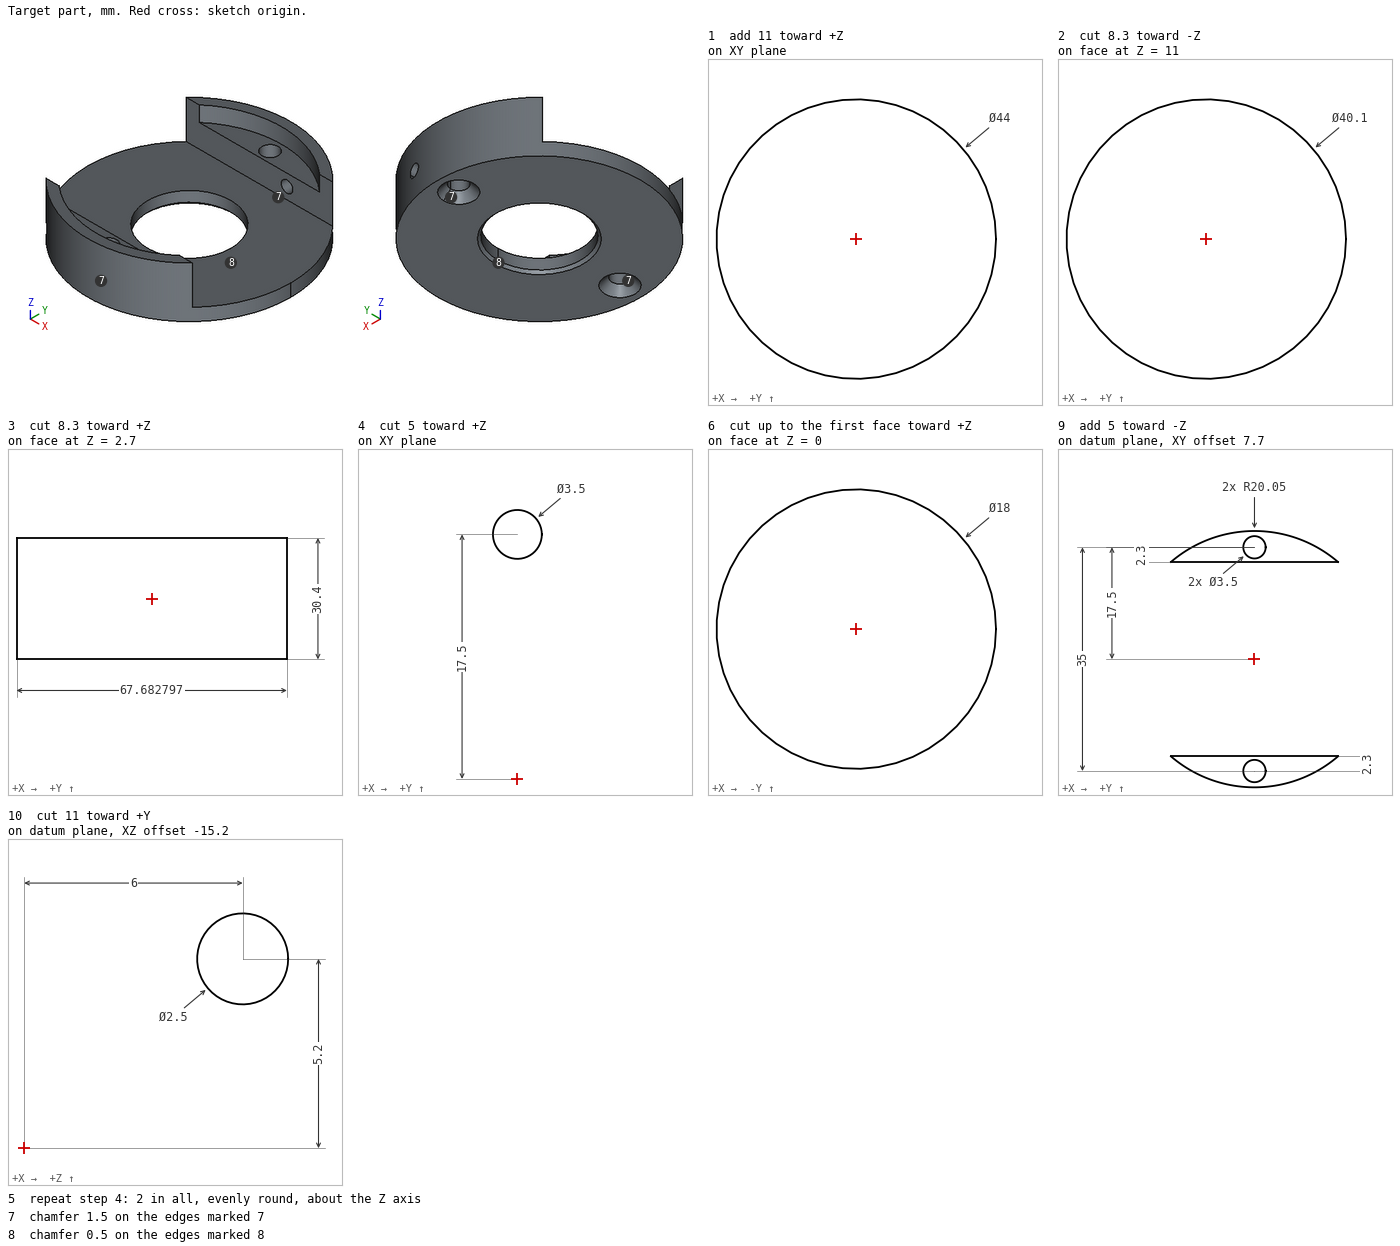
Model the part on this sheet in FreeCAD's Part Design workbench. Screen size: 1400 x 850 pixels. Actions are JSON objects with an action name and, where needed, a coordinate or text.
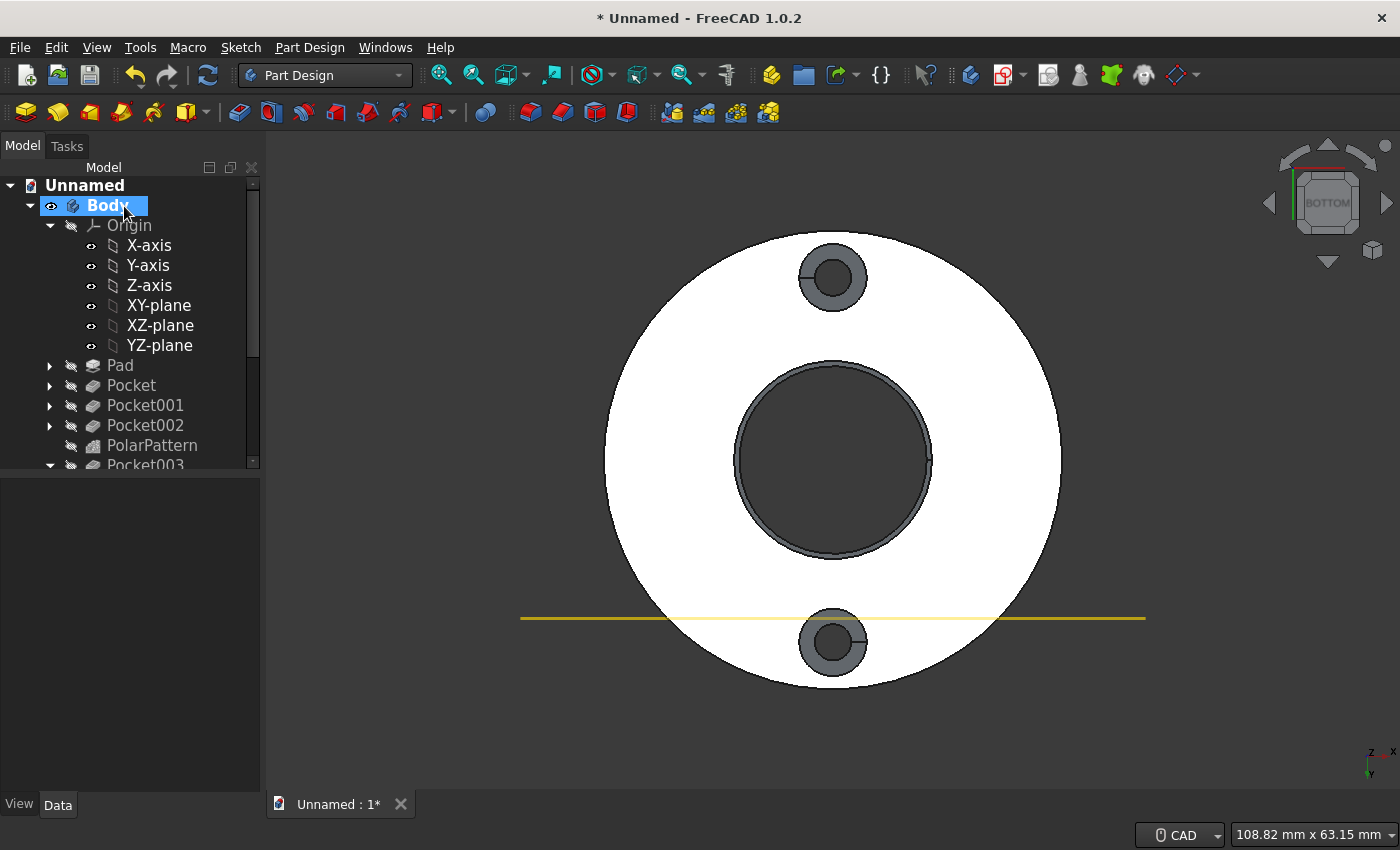
{"action": "scroll", "coordinate": [100, 321], "scroll_direction": "down", "scroll_amount": 3}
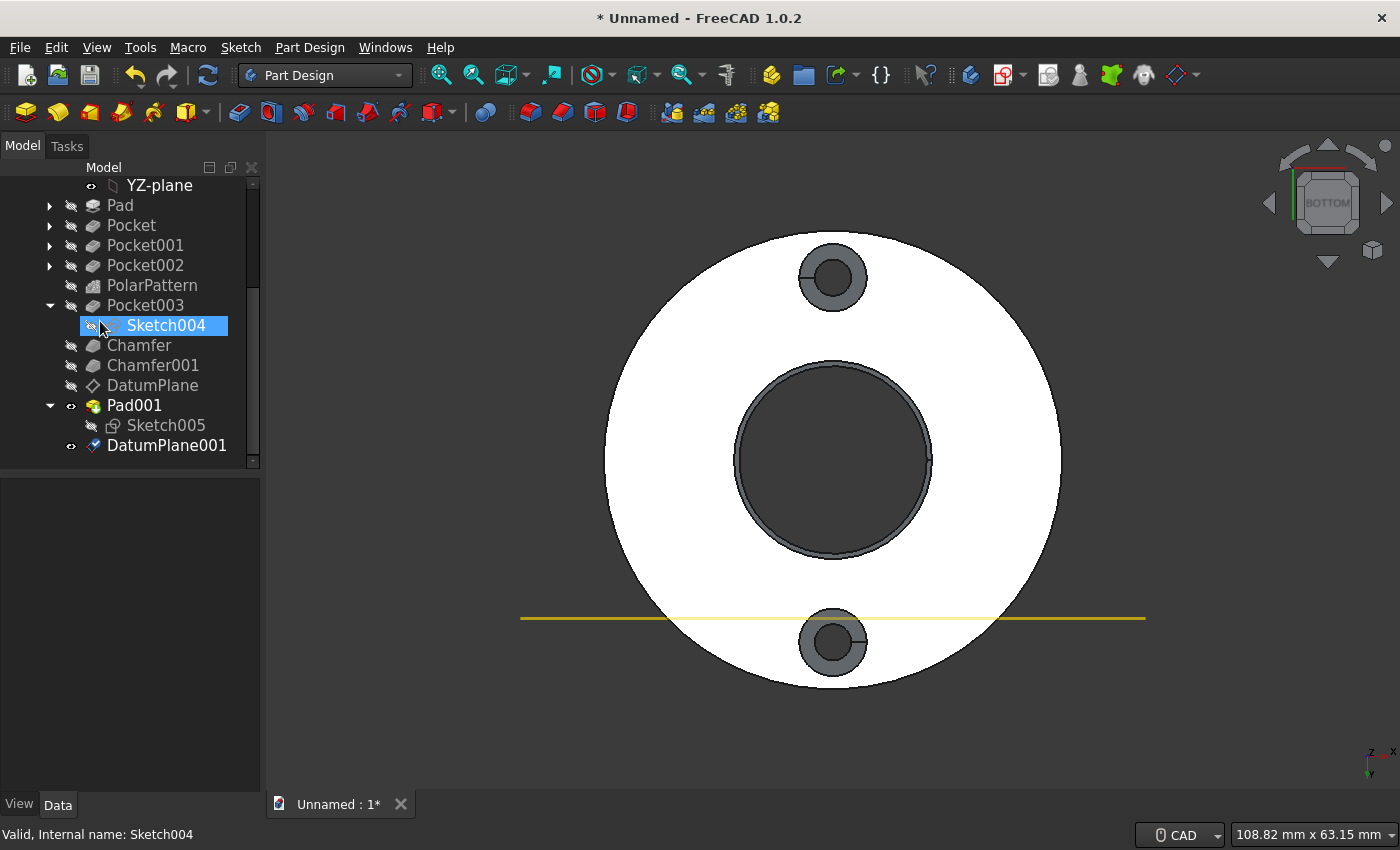
{"action": "left_click", "coordinate": [116, 446]}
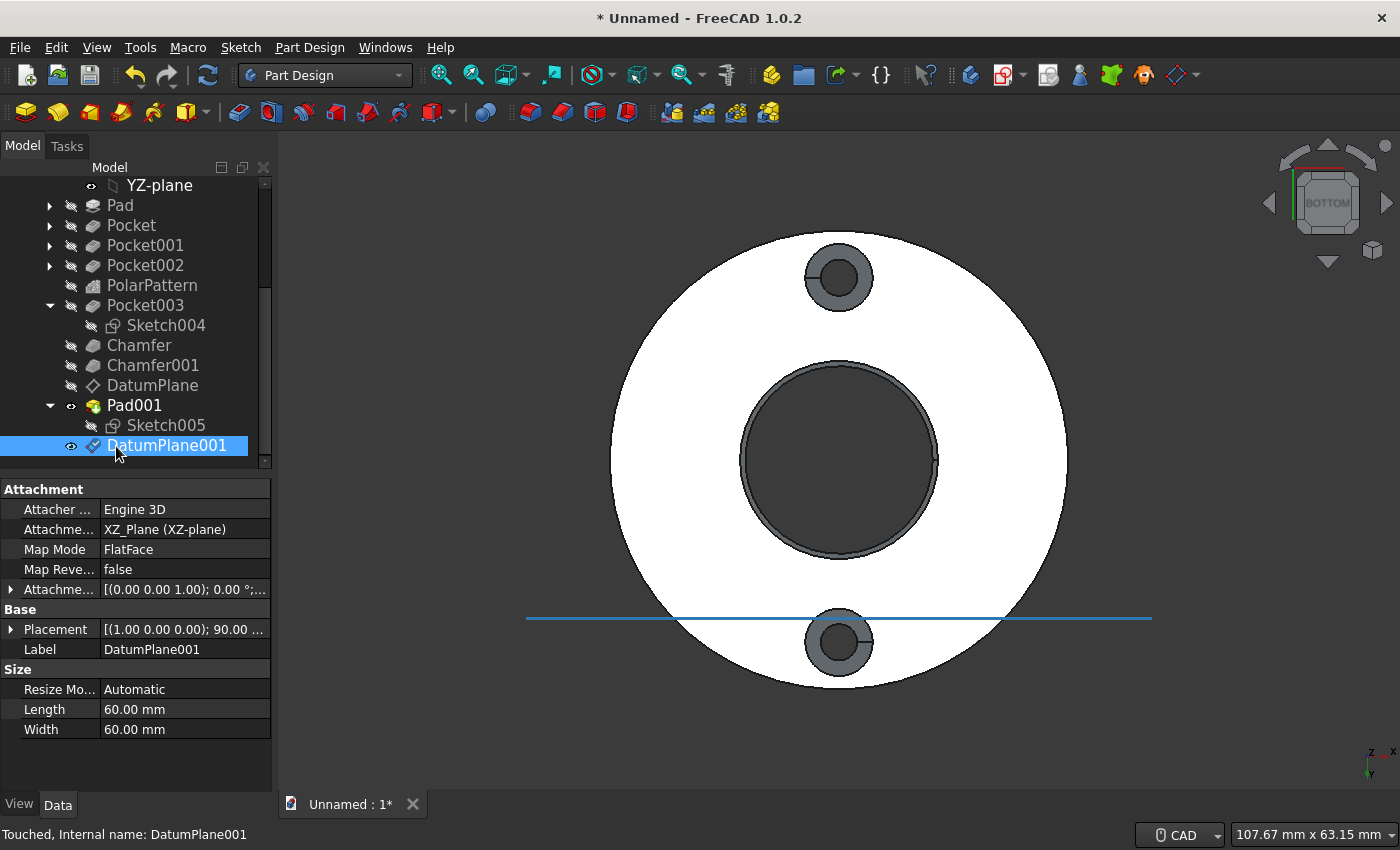
{"action": "left_click", "coordinate": [1004, 76]}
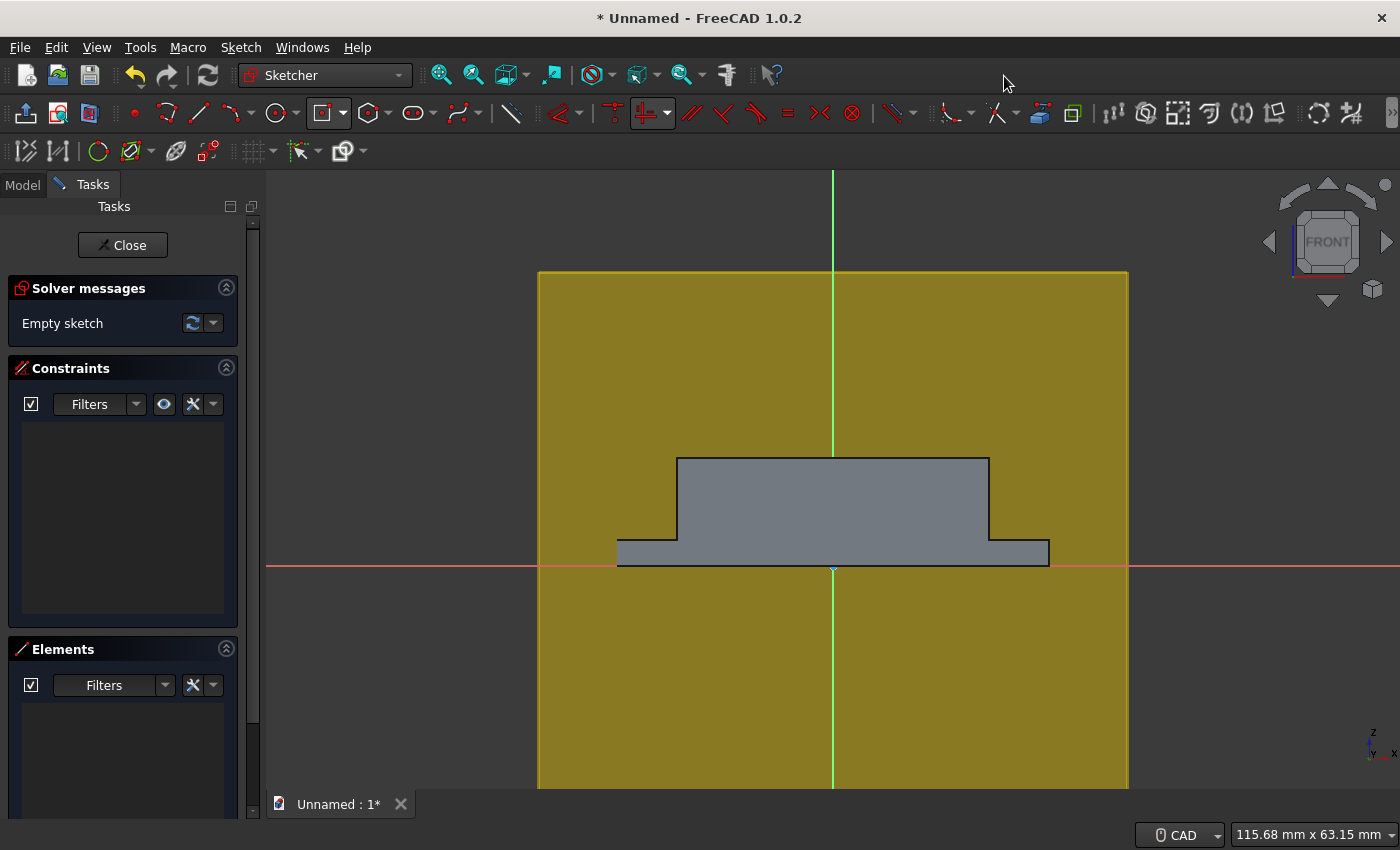
{"action": "left_click", "coordinate": [90, 114]}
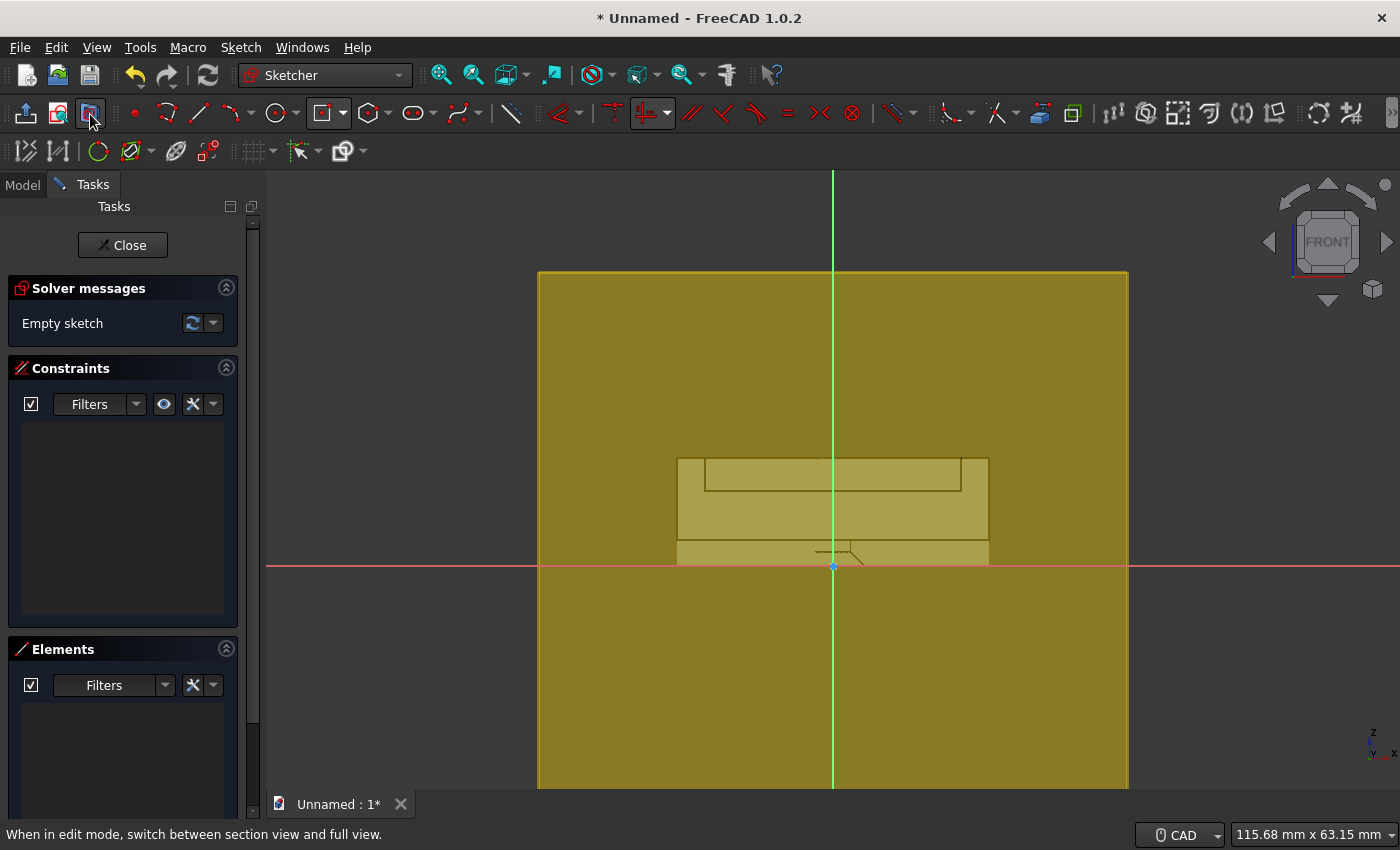
{"action": "scroll", "coordinate": [900, 518], "scroll_direction": "up", "scroll_amount": 14}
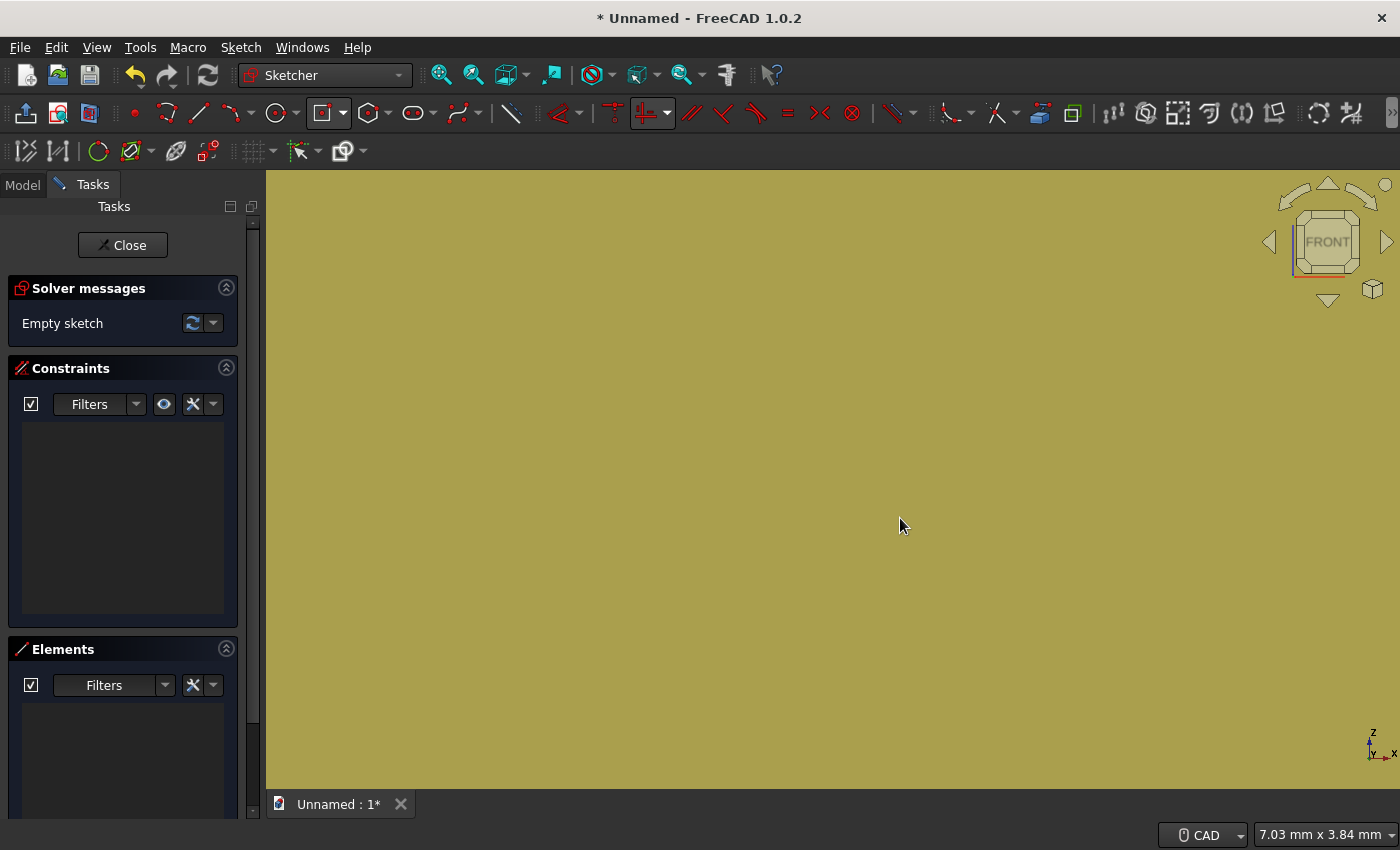
{"action": "left_click", "coordinate": [276, 114]}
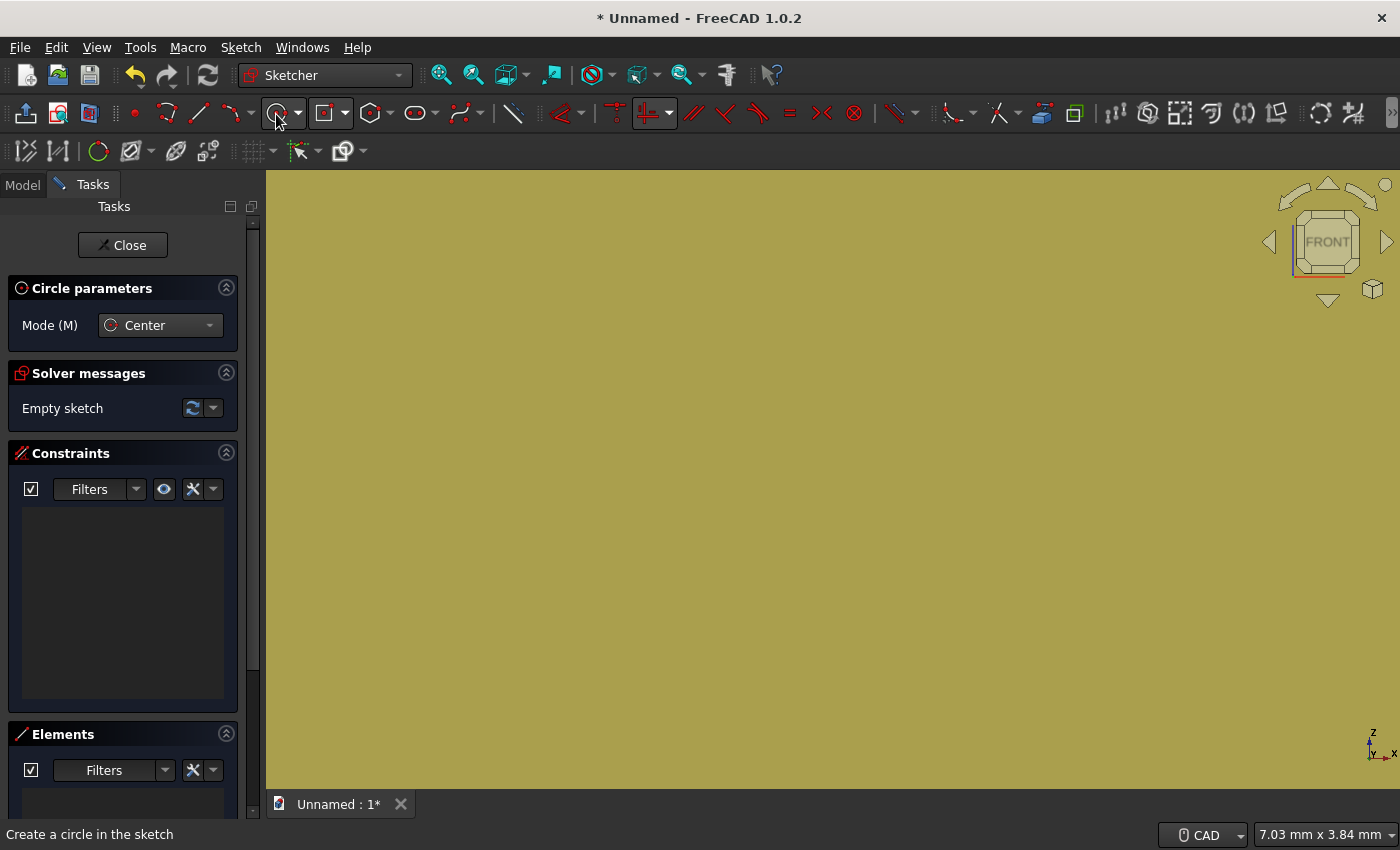
{"action": "left_click", "coordinate": [757, 465]}
{"action": "left_click", "coordinate": [899, 322]}
{"action": "key", "text": "Escape"}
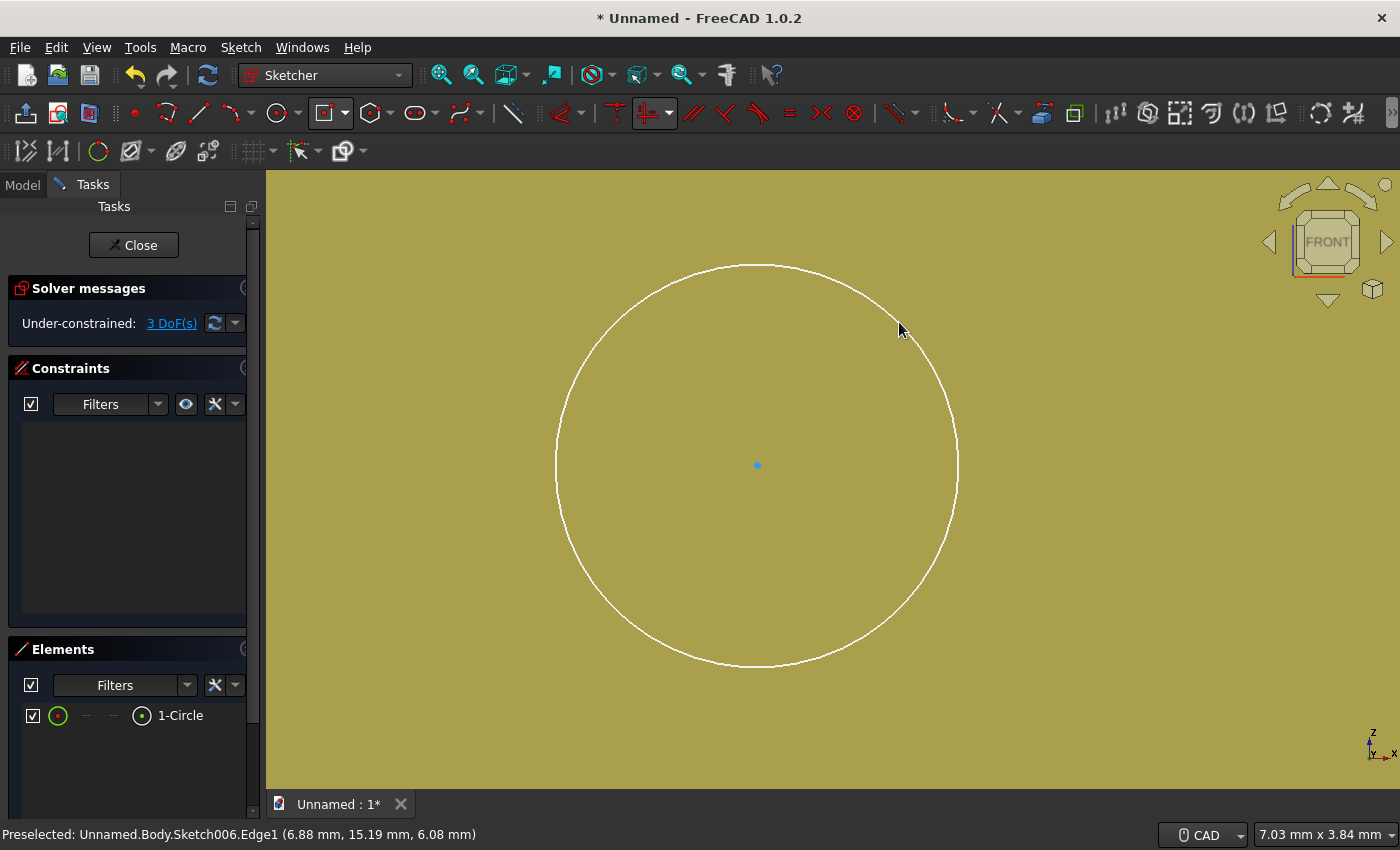
{"action": "key", "text": "d"}